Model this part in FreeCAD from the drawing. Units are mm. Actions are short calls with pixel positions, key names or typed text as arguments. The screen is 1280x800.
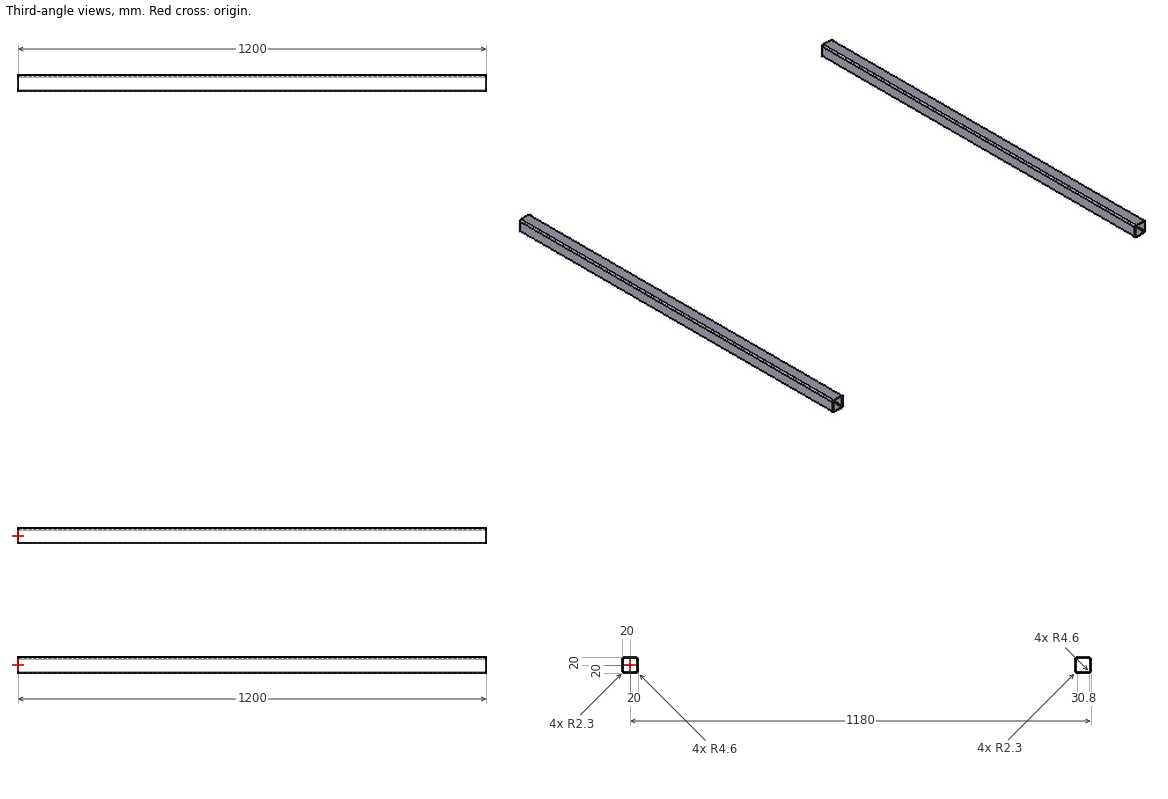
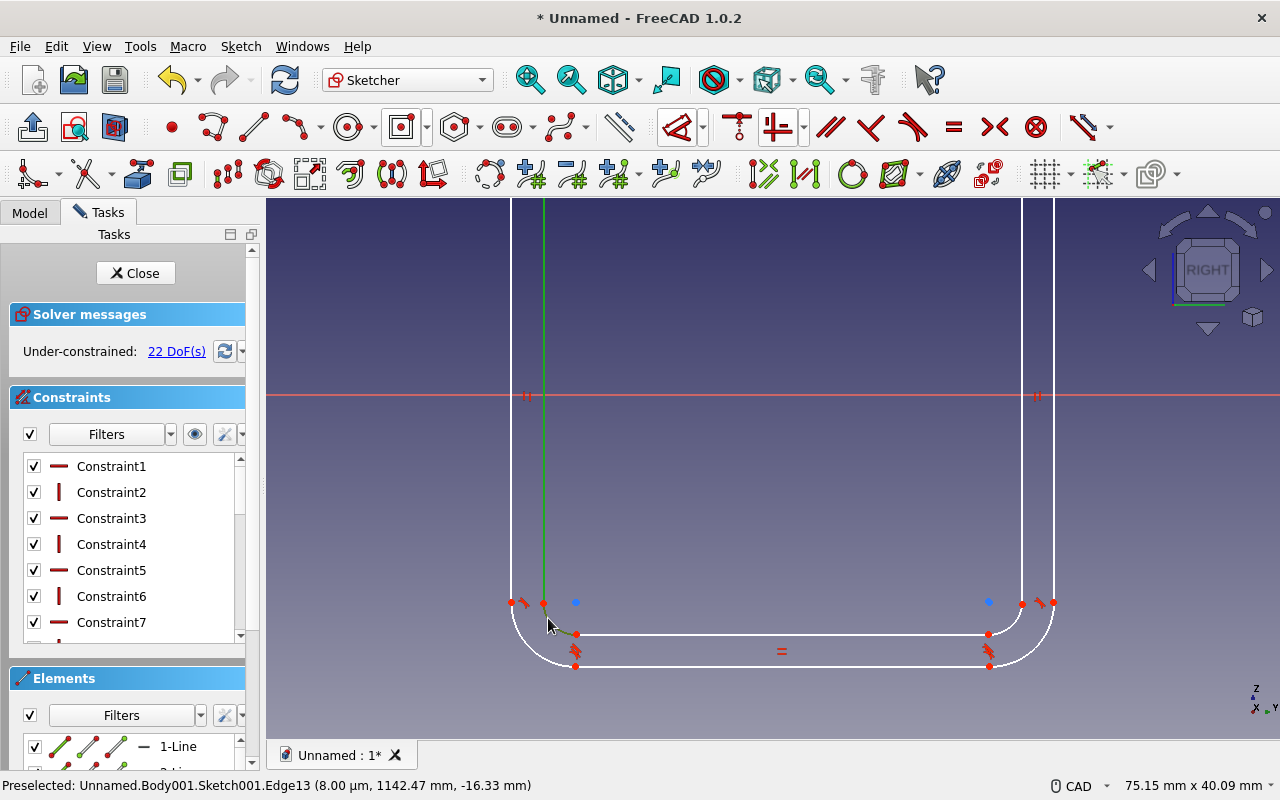
key(t)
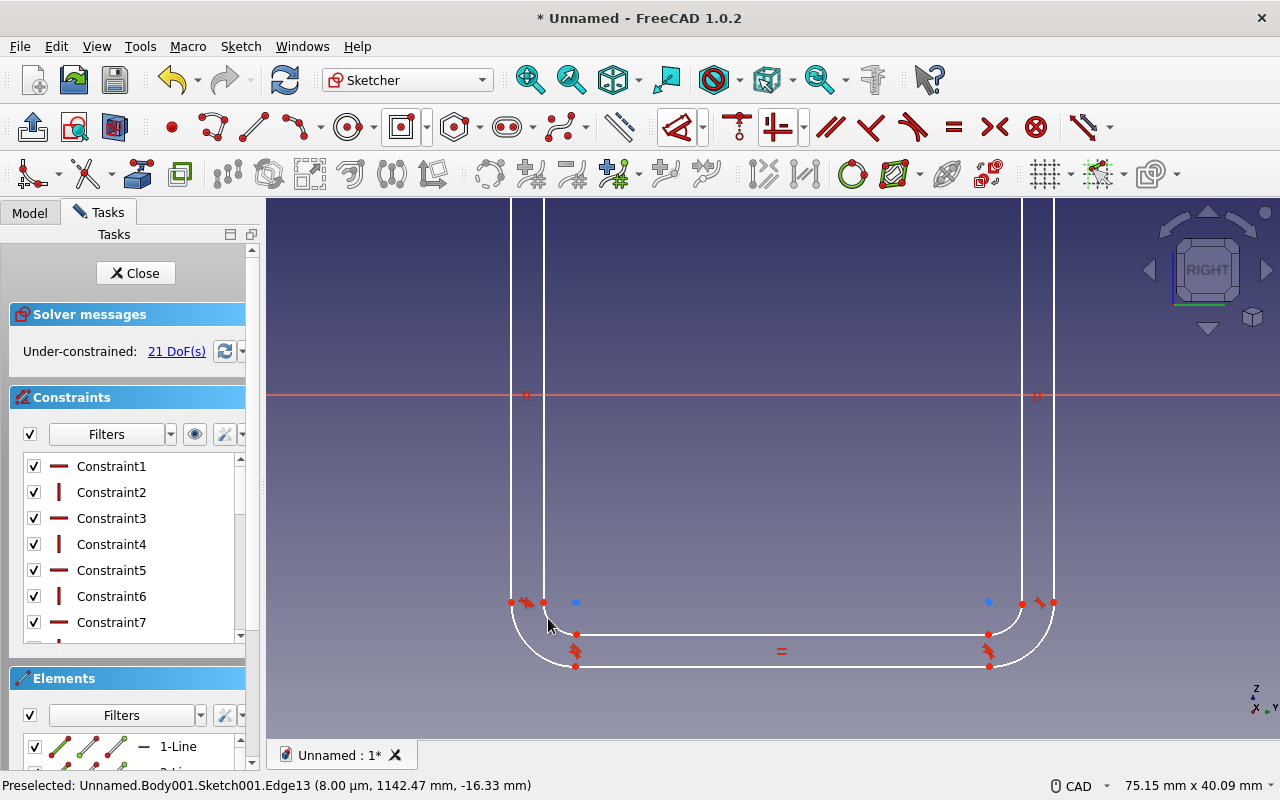
click(544, 478)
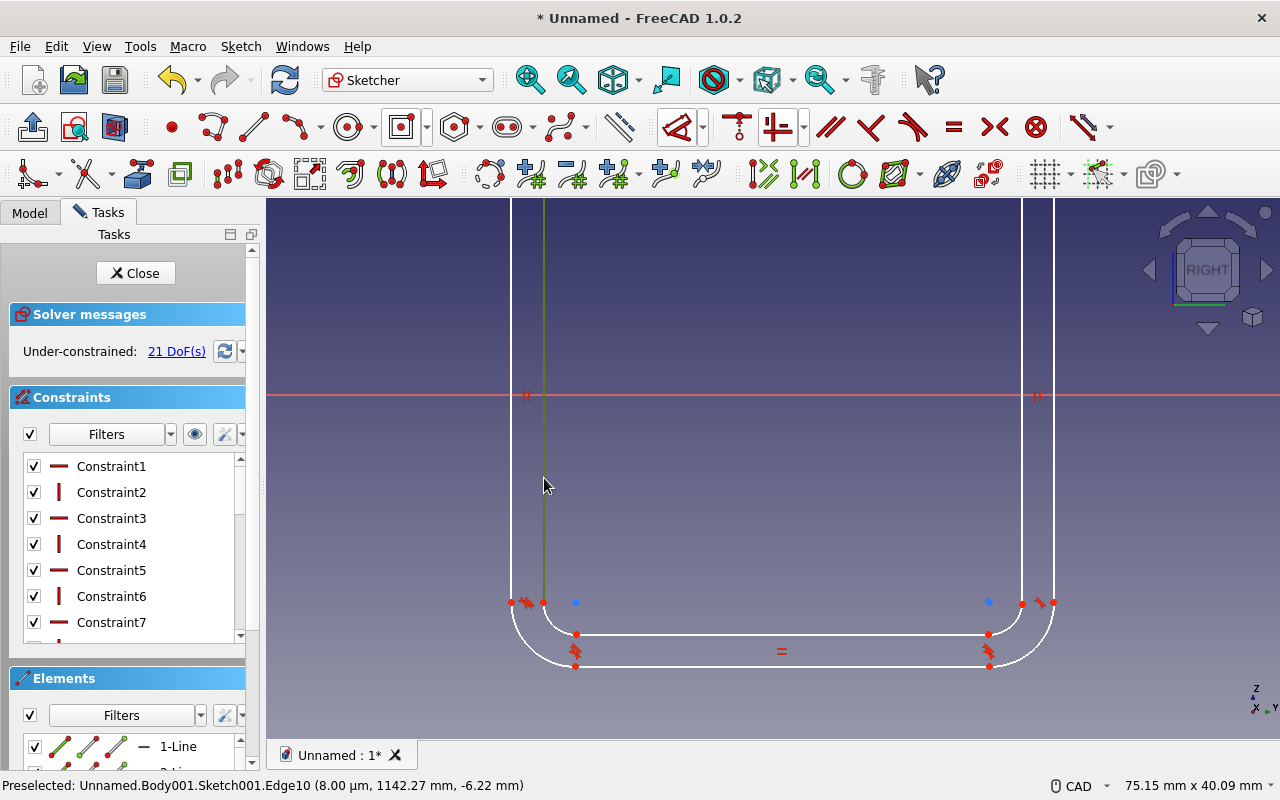
scroll(545, 618, down, 2)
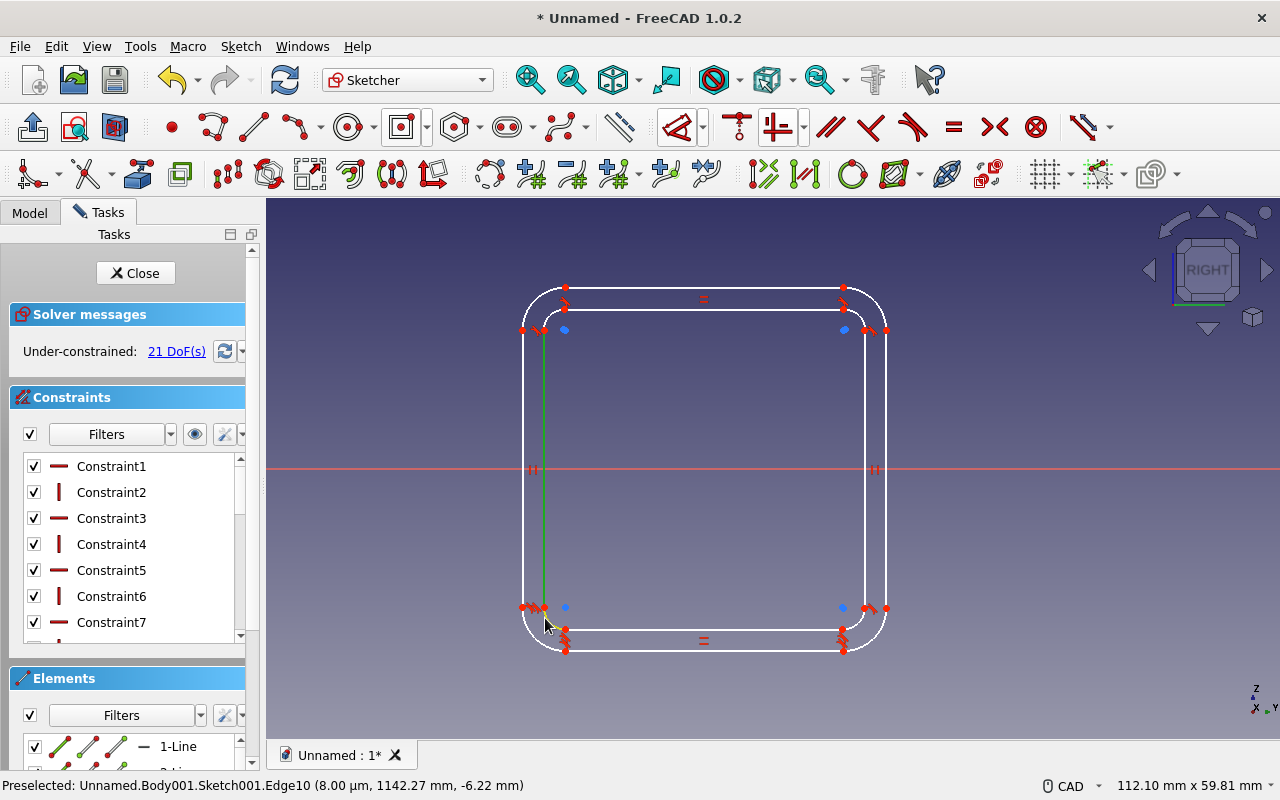
scroll(555, 312, up, 2)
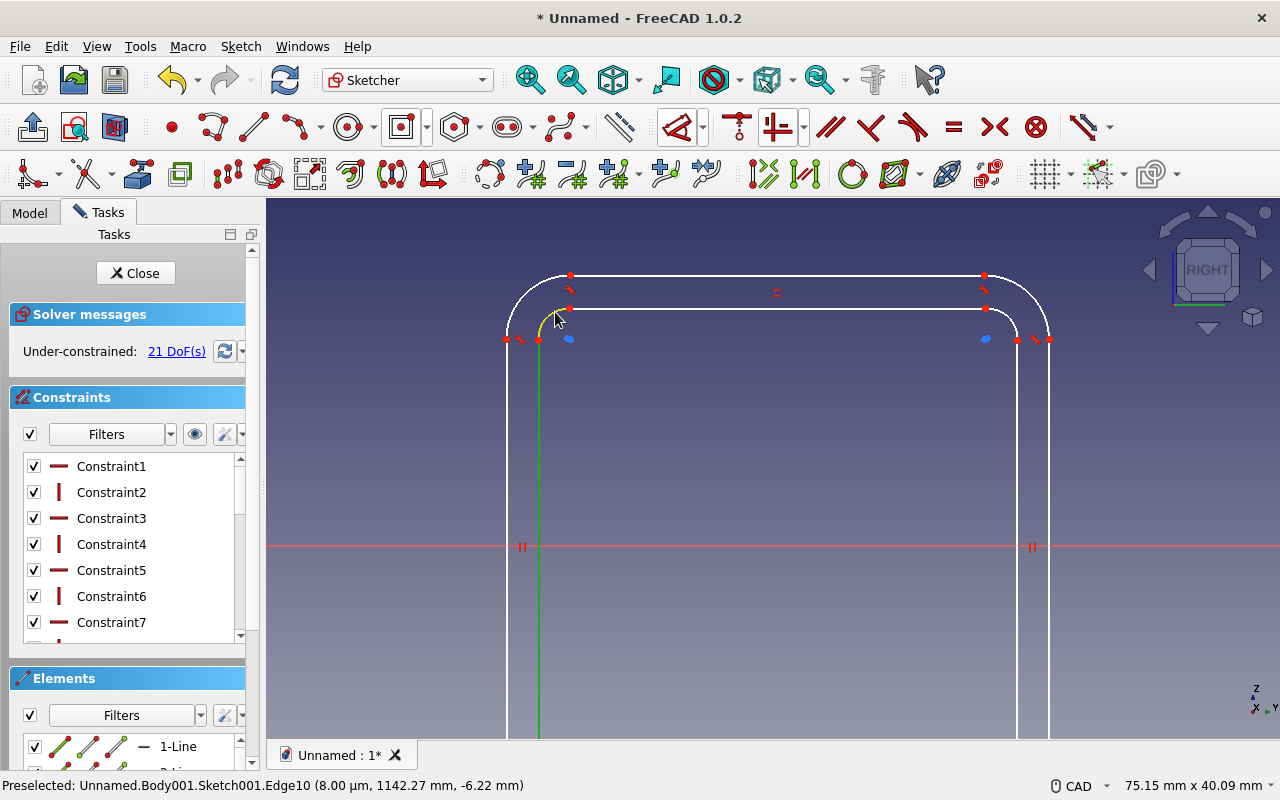
click(555, 312)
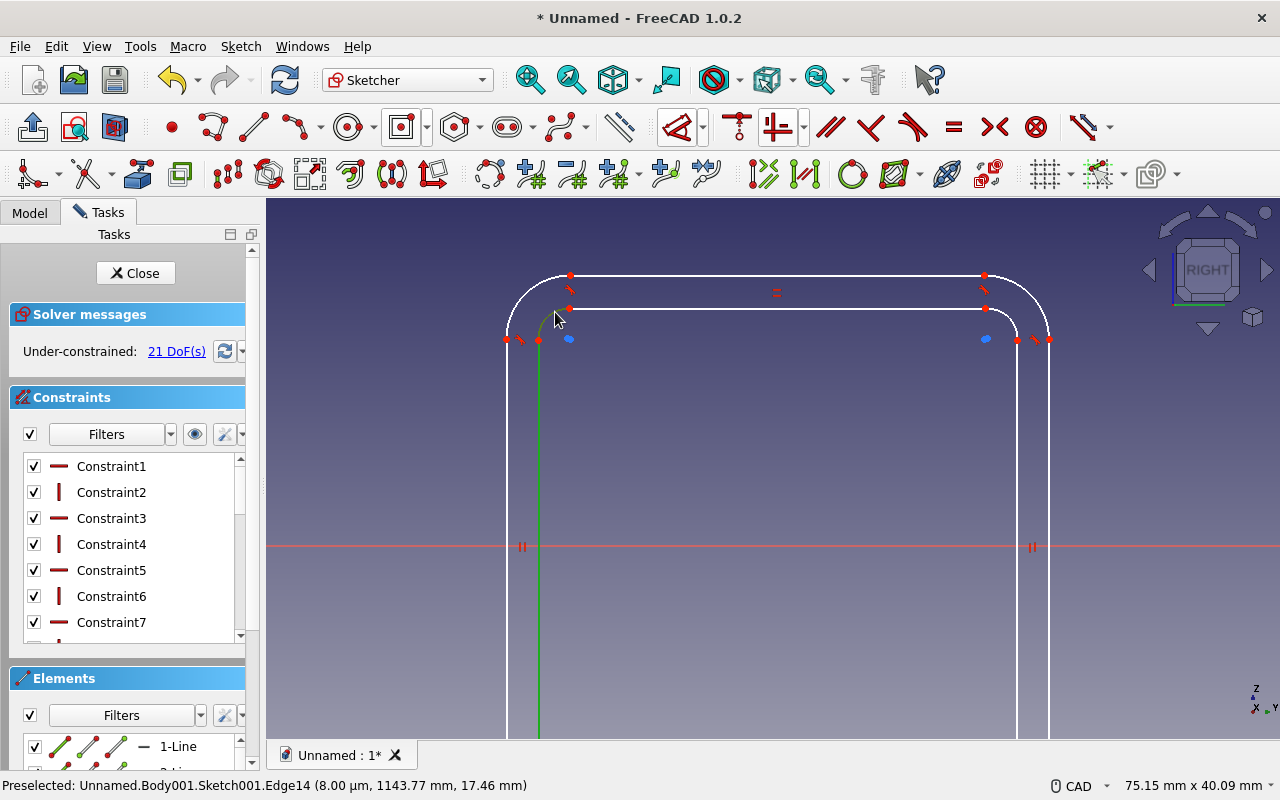
key(t)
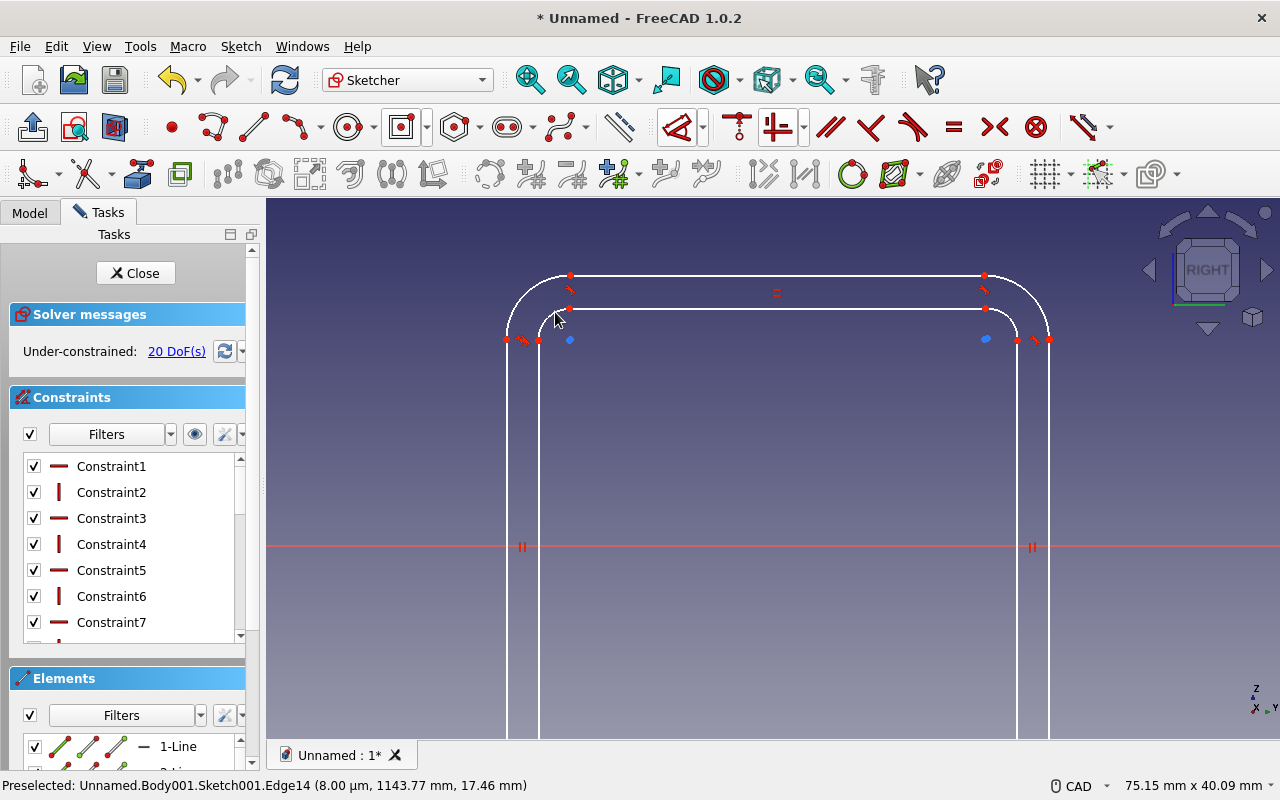
click(695, 309)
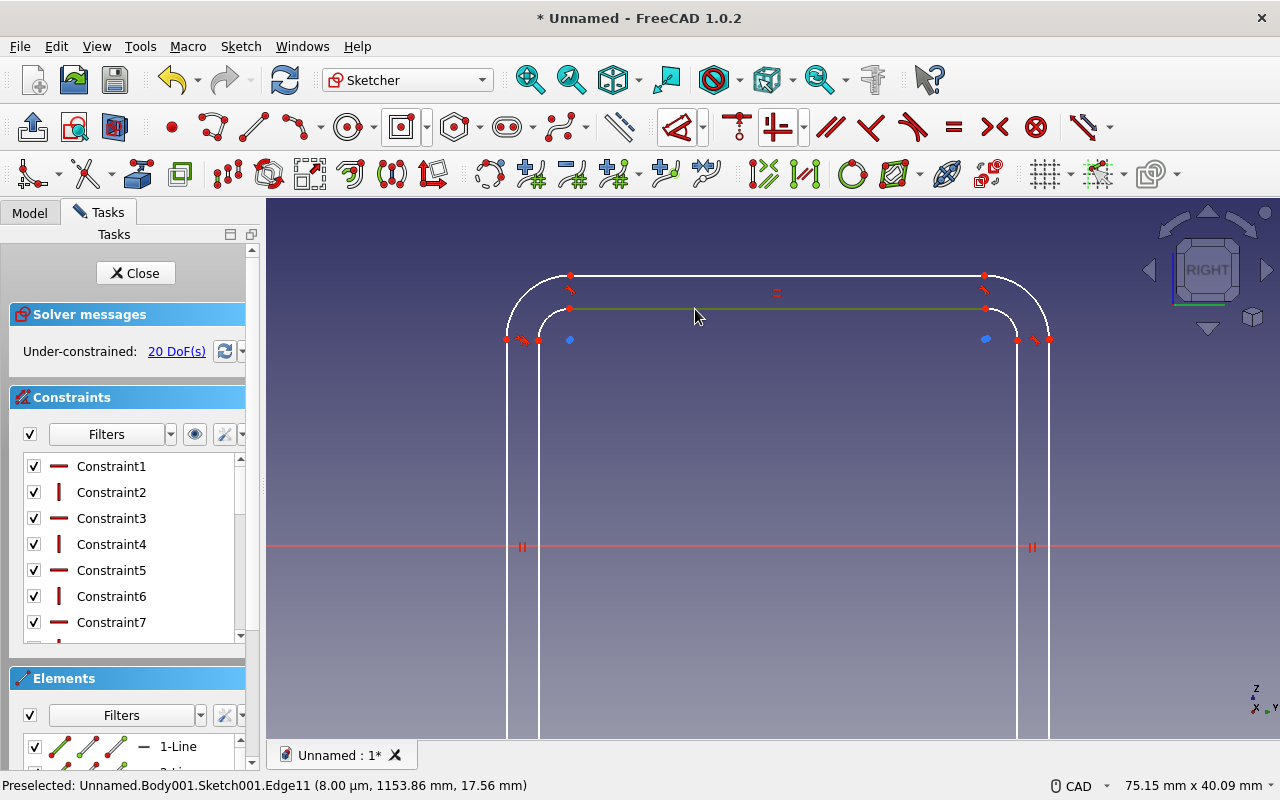
click(556, 312)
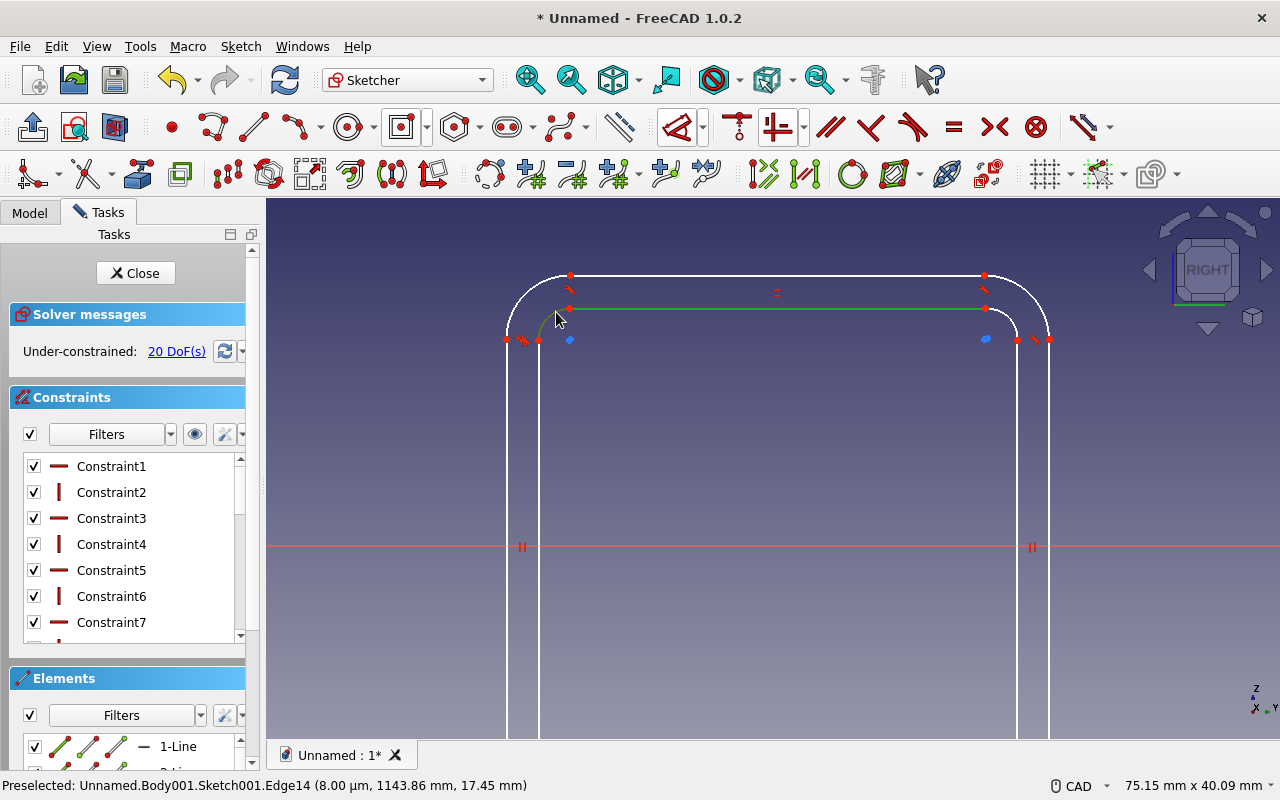
key(t)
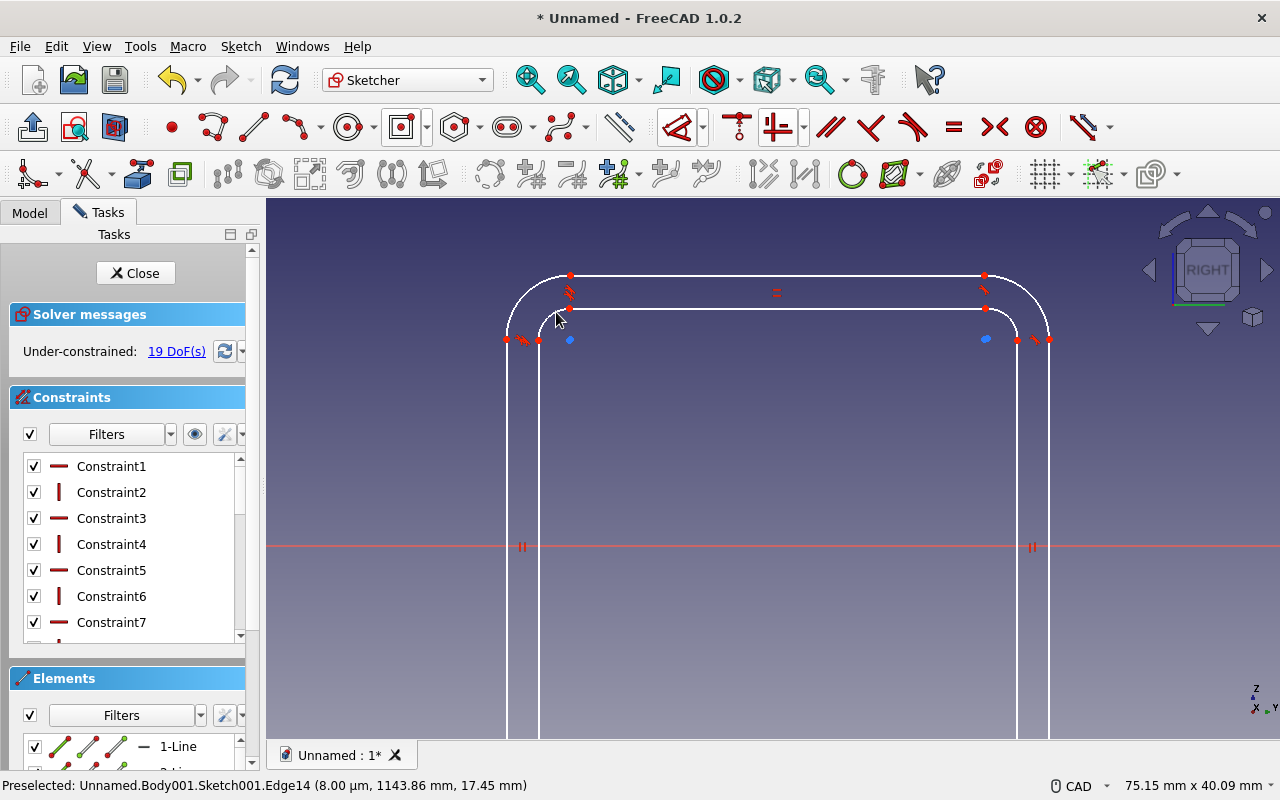
click(695, 309)